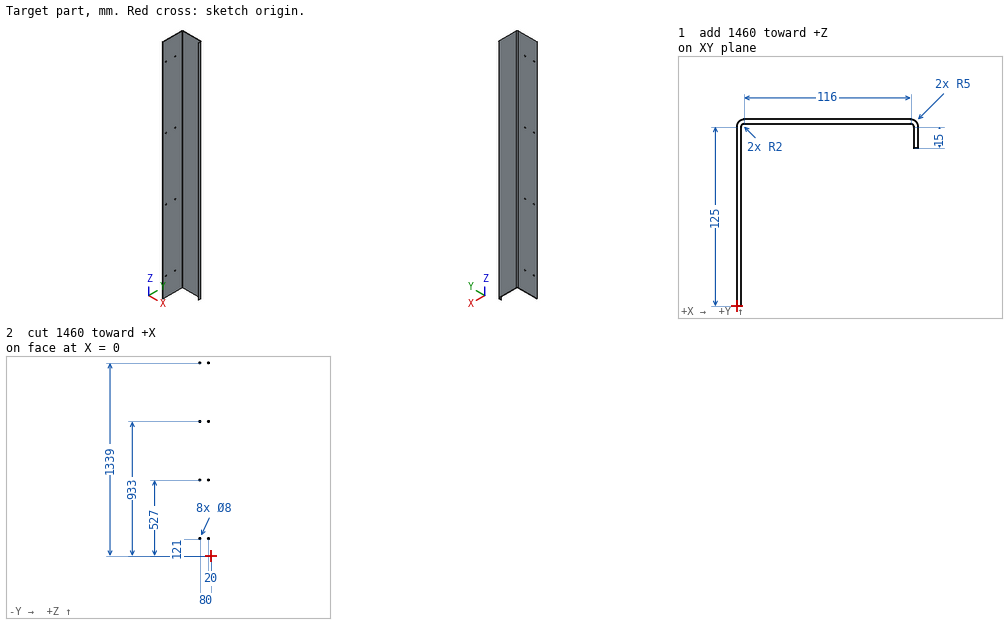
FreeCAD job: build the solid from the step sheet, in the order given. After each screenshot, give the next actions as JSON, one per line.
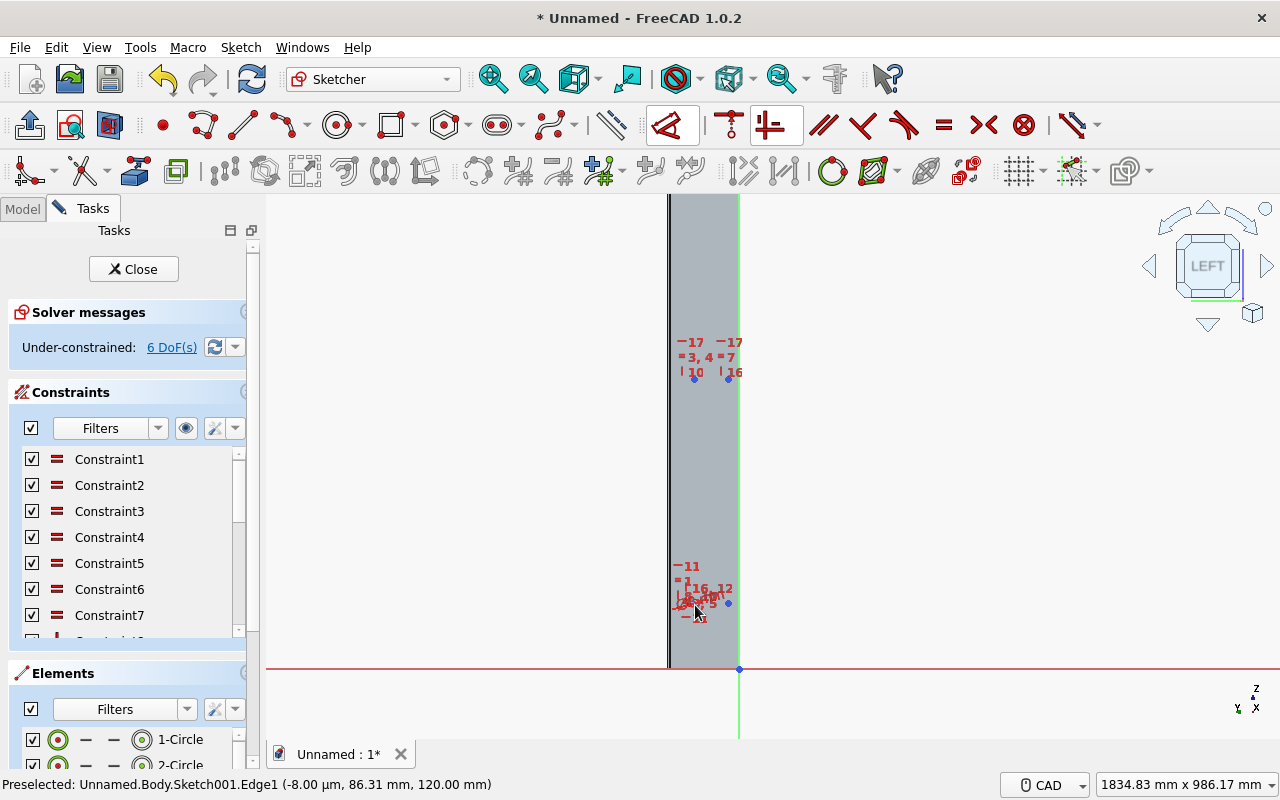
{"action": "left_click", "coordinate": [695, 603]}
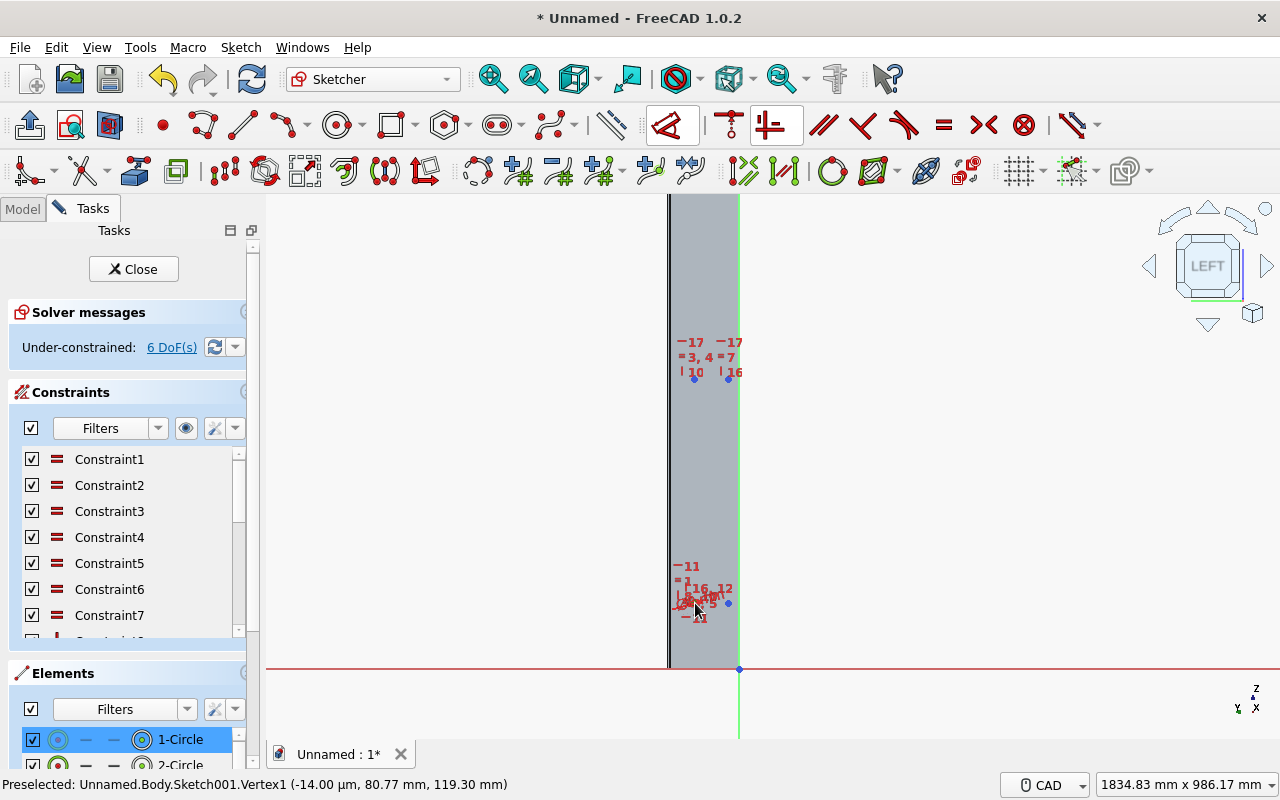
{"action": "key", "text": "l"}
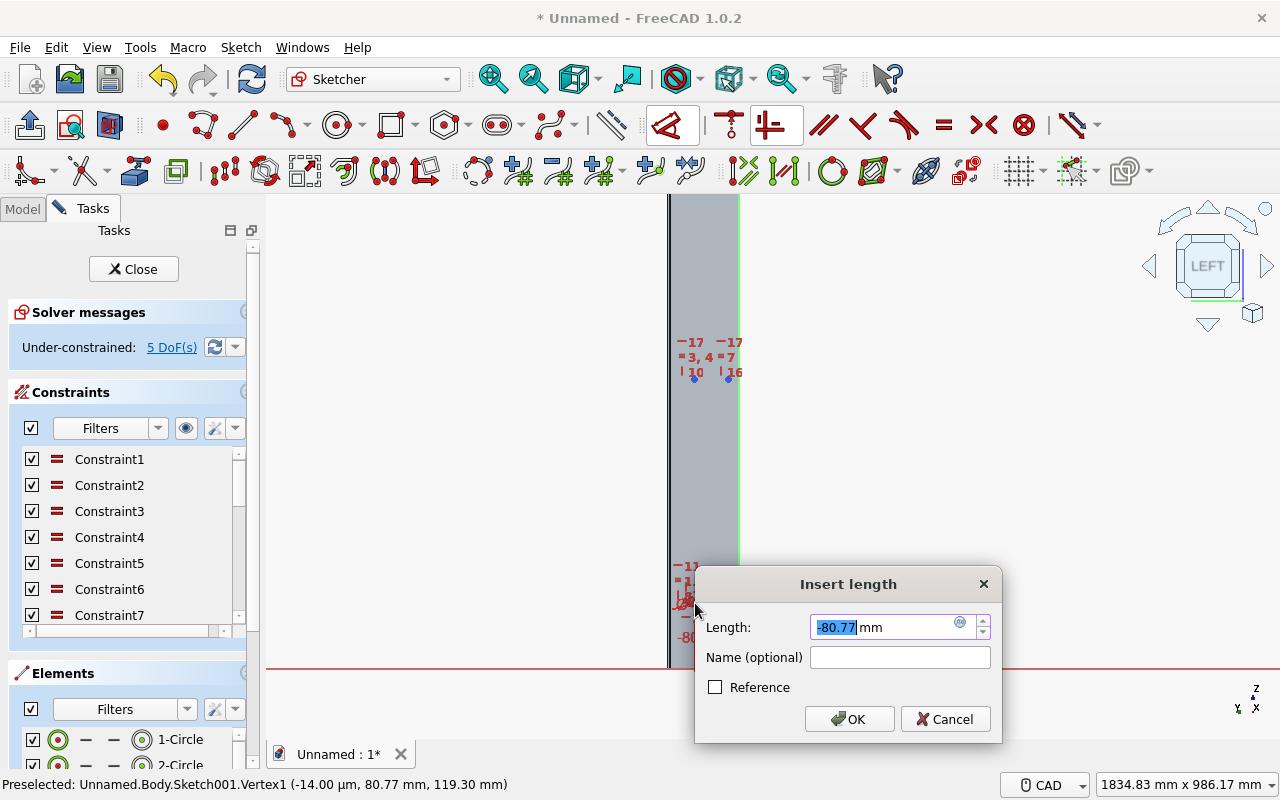
{"action": "type", "text": "-80"}
{"action": "key", "text": "Return"}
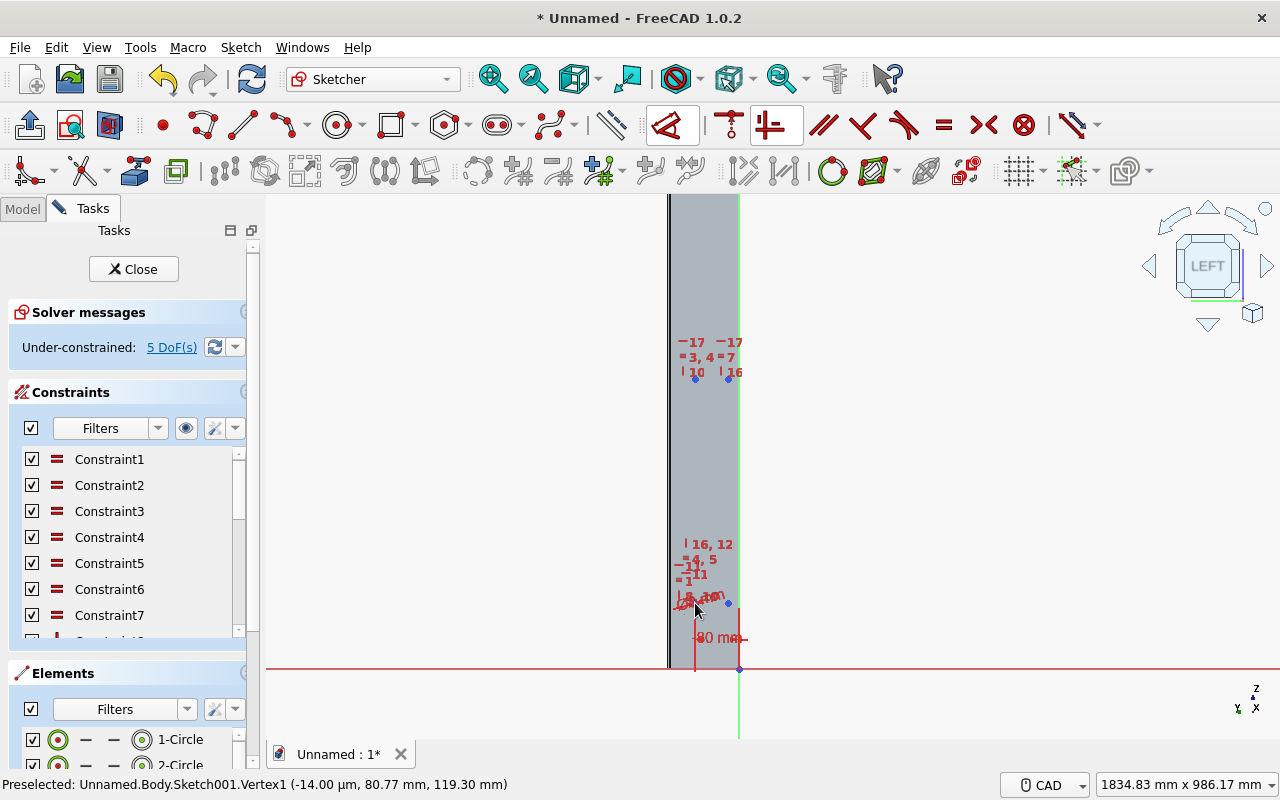
{"action": "scroll", "coordinate": [728, 603], "scroll_direction": "up", "scroll_amount": 7}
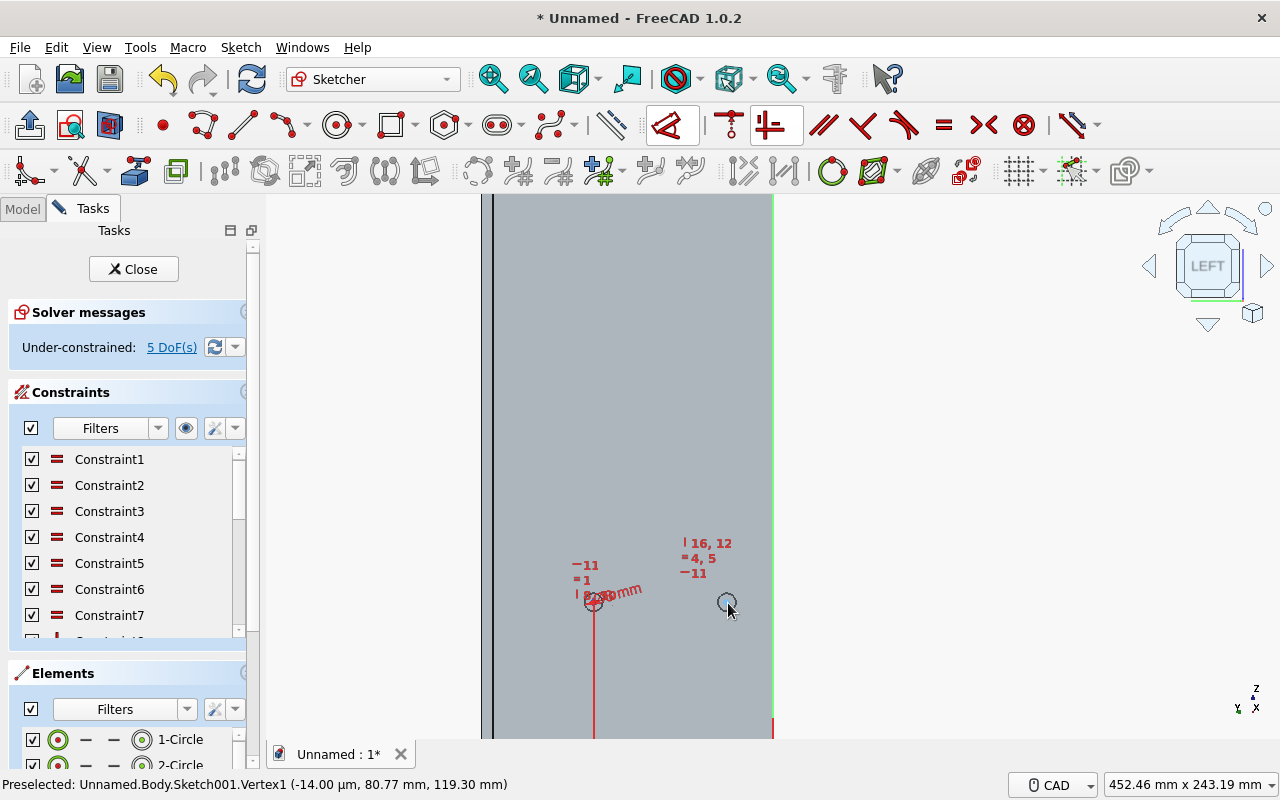
{"action": "left_click", "coordinate": [727, 602]}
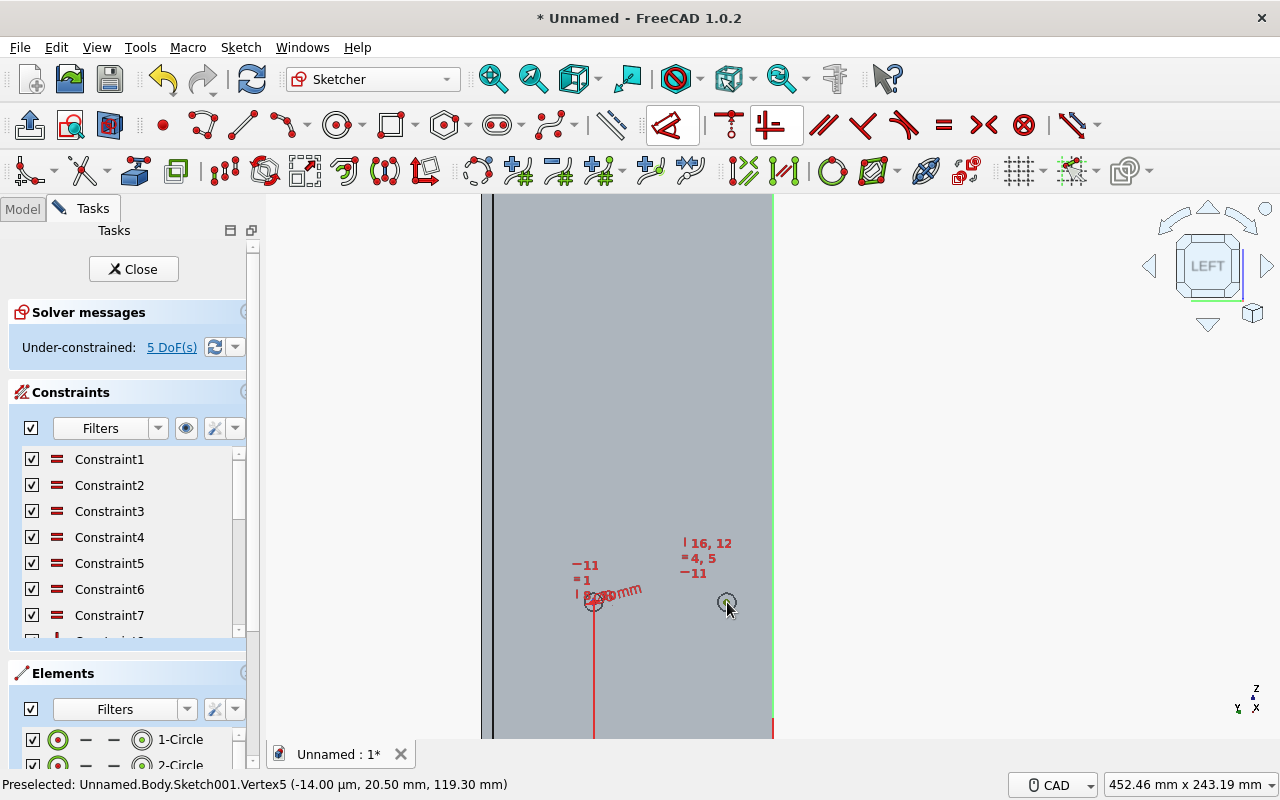
{"action": "key", "text": "l"}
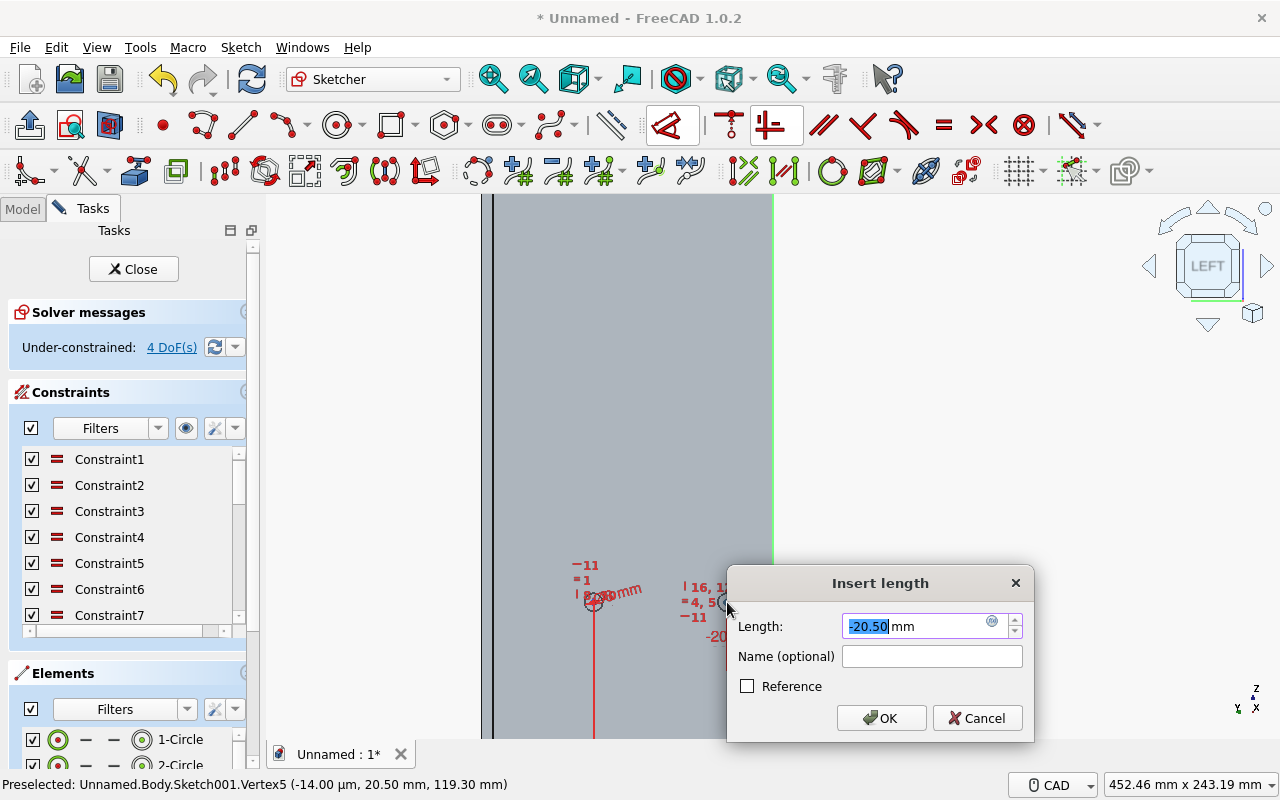
{"action": "type", "text": "-20"}
{"action": "key", "text": "Return"}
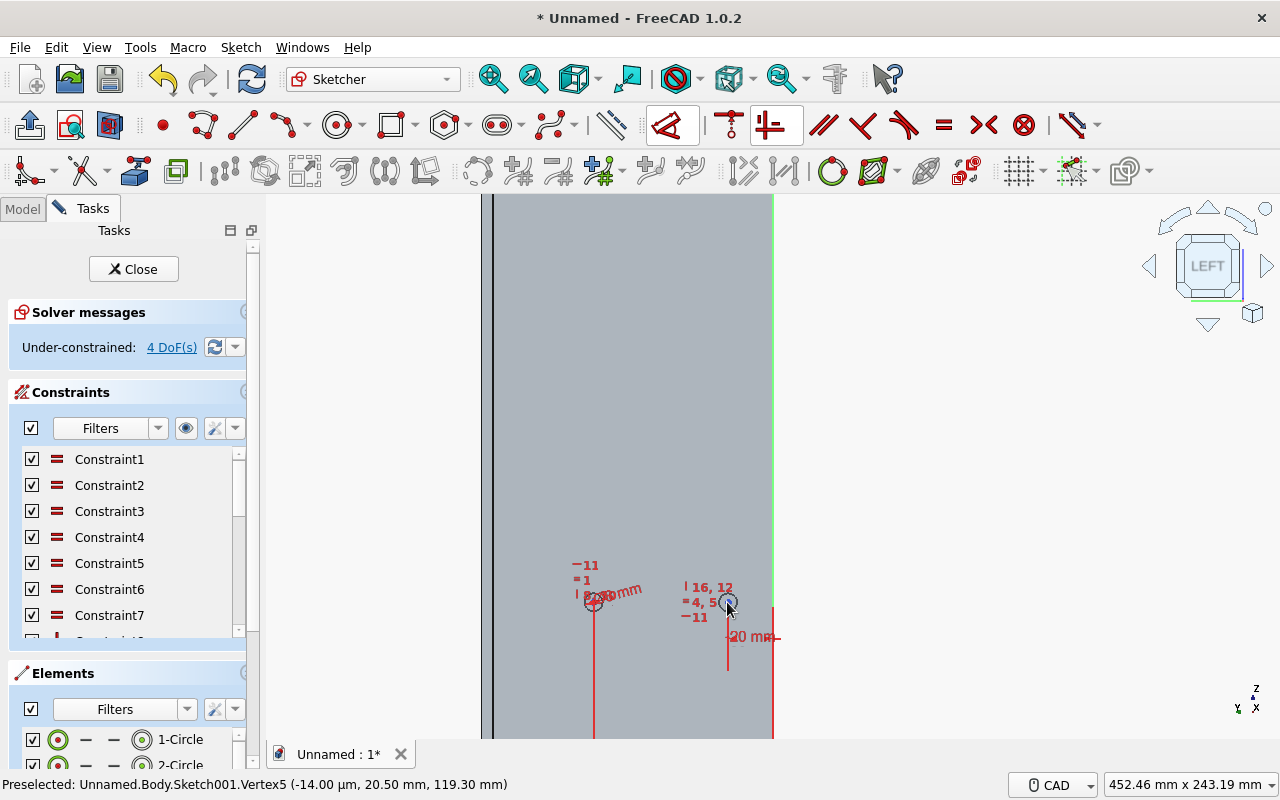
{"action": "scroll", "coordinate": [708, 604], "scroll_direction": "down", "scroll_amount": 11}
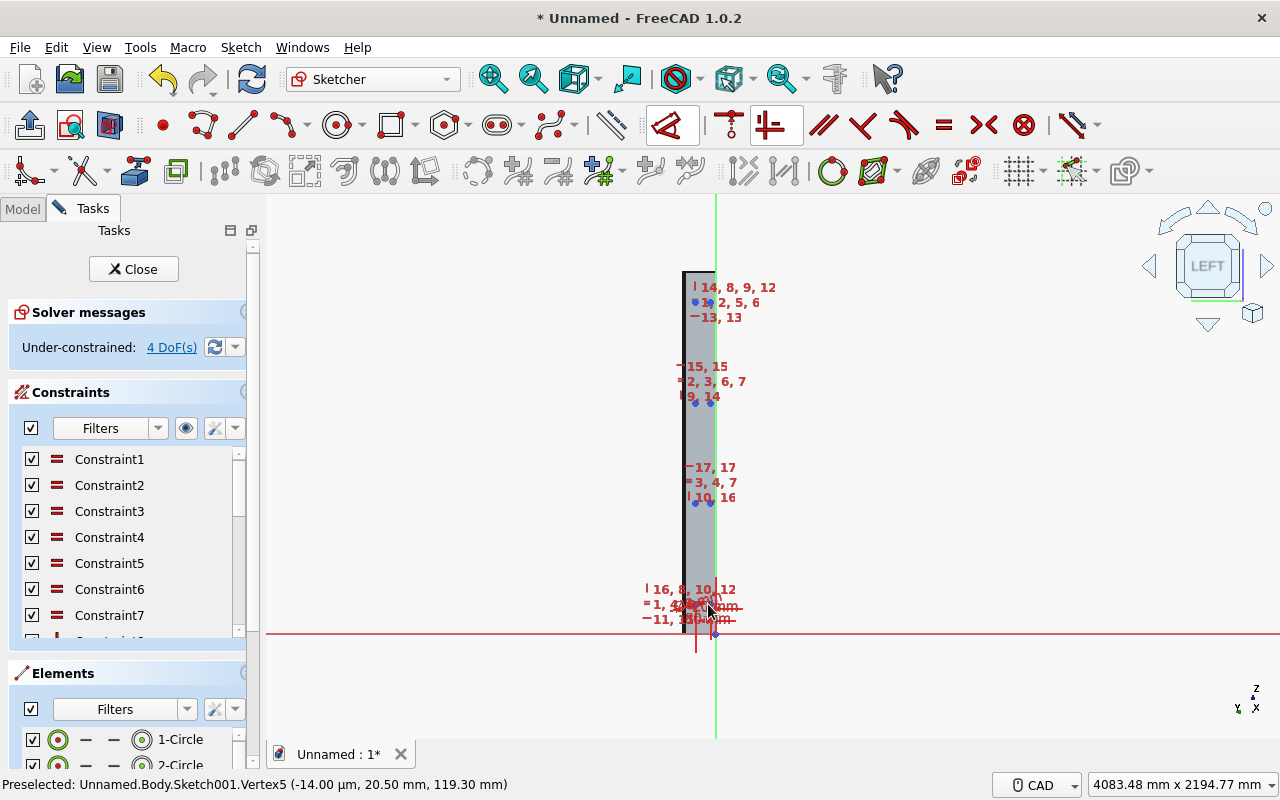
{"action": "scroll", "coordinate": [696, 604], "scroll_direction": "up", "scroll_amount": 2}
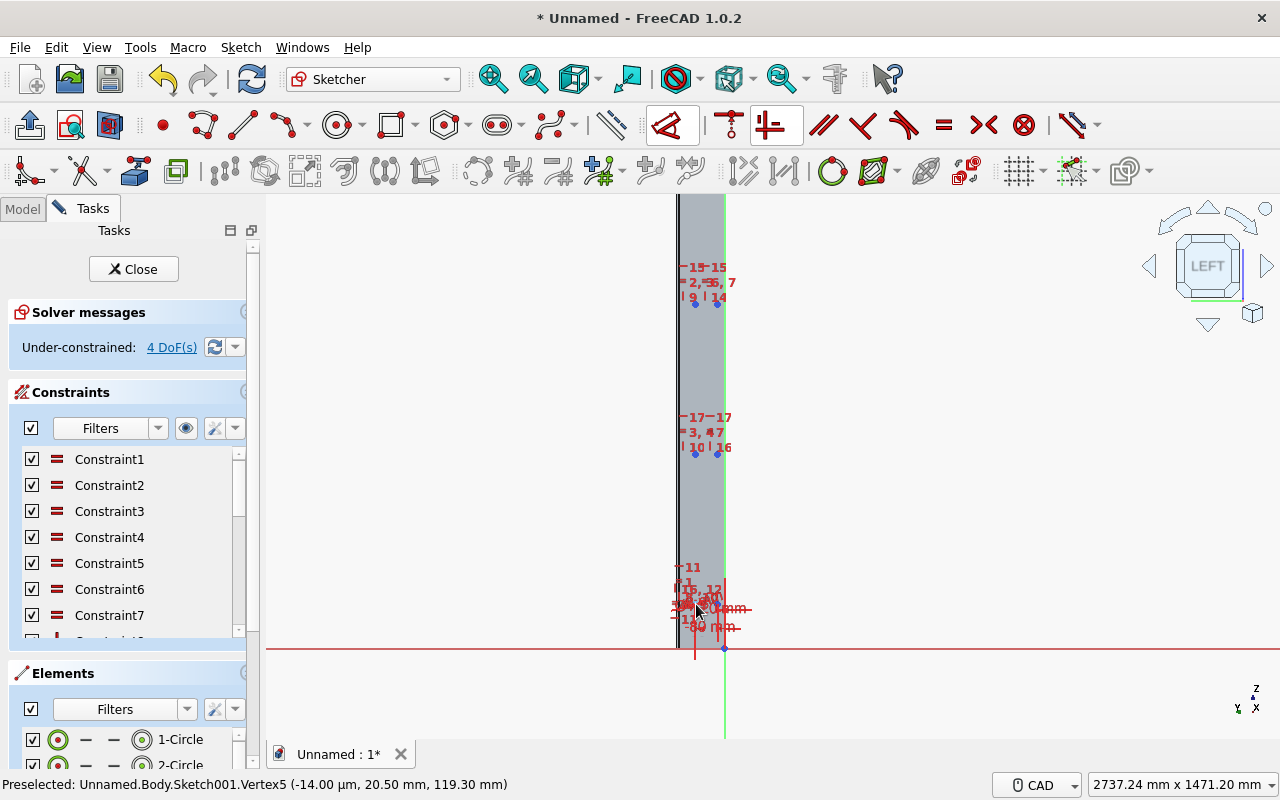
{"action": "left_click", "coordinate": [695, 604]}